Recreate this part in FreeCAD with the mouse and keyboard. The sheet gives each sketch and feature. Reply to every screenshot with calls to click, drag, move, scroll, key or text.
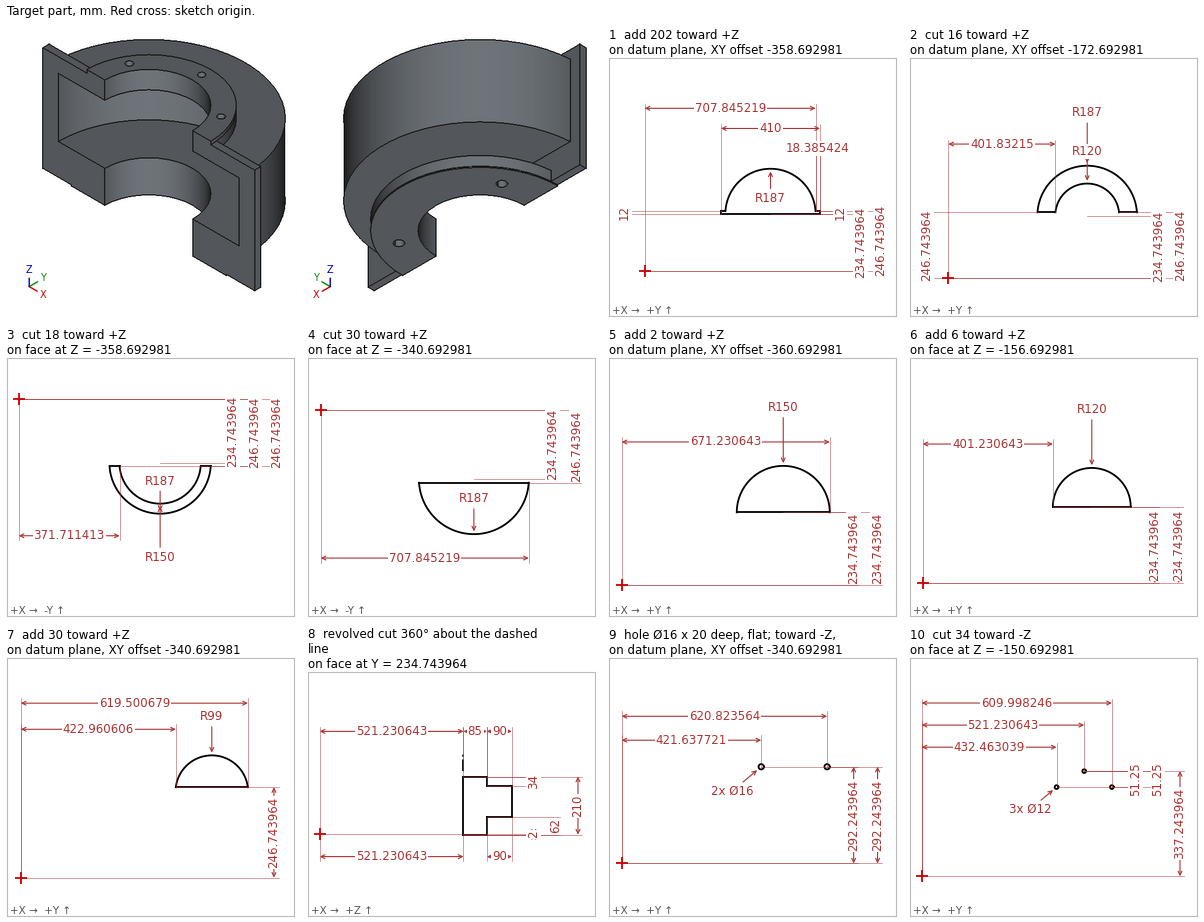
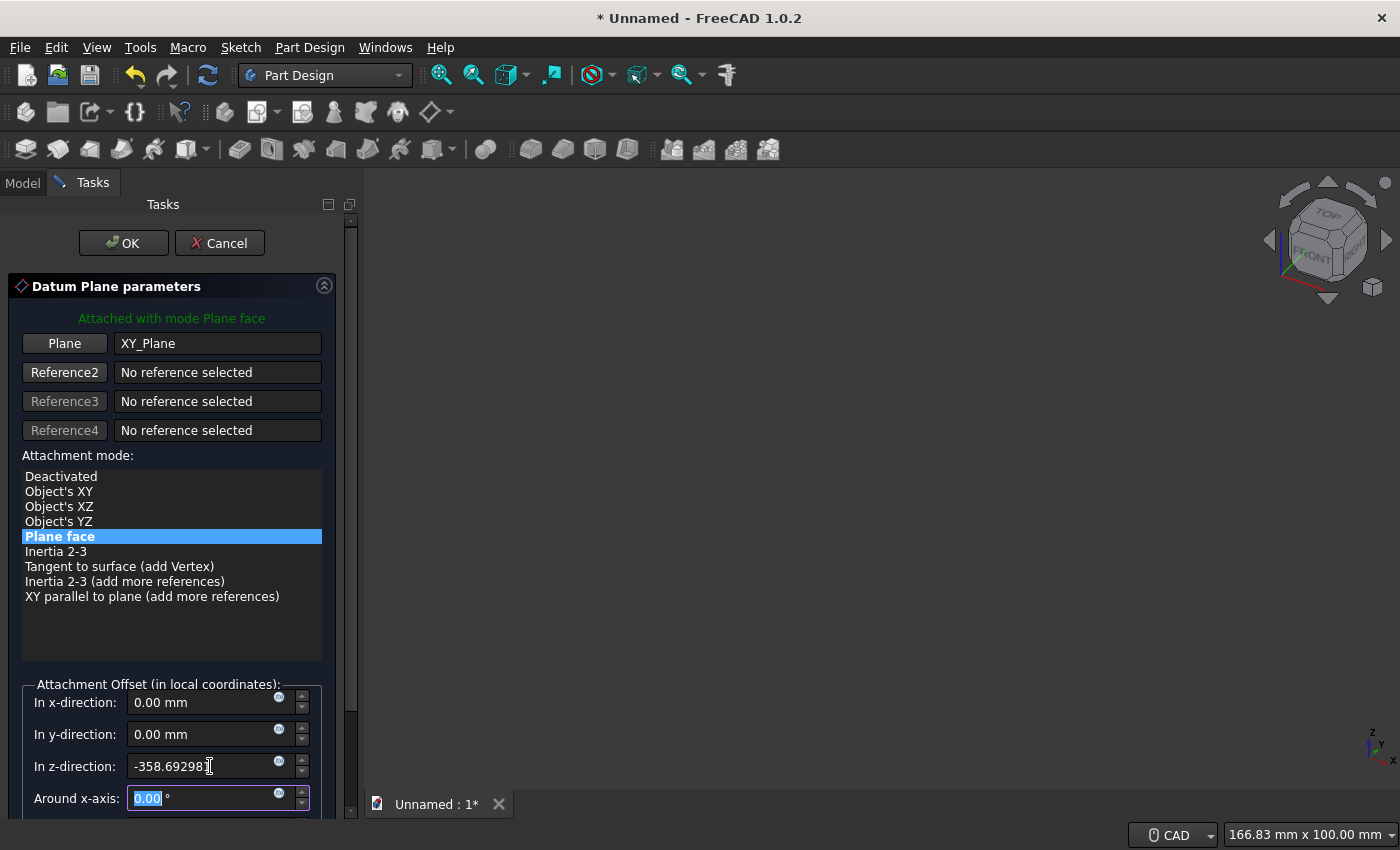
click(124, 243)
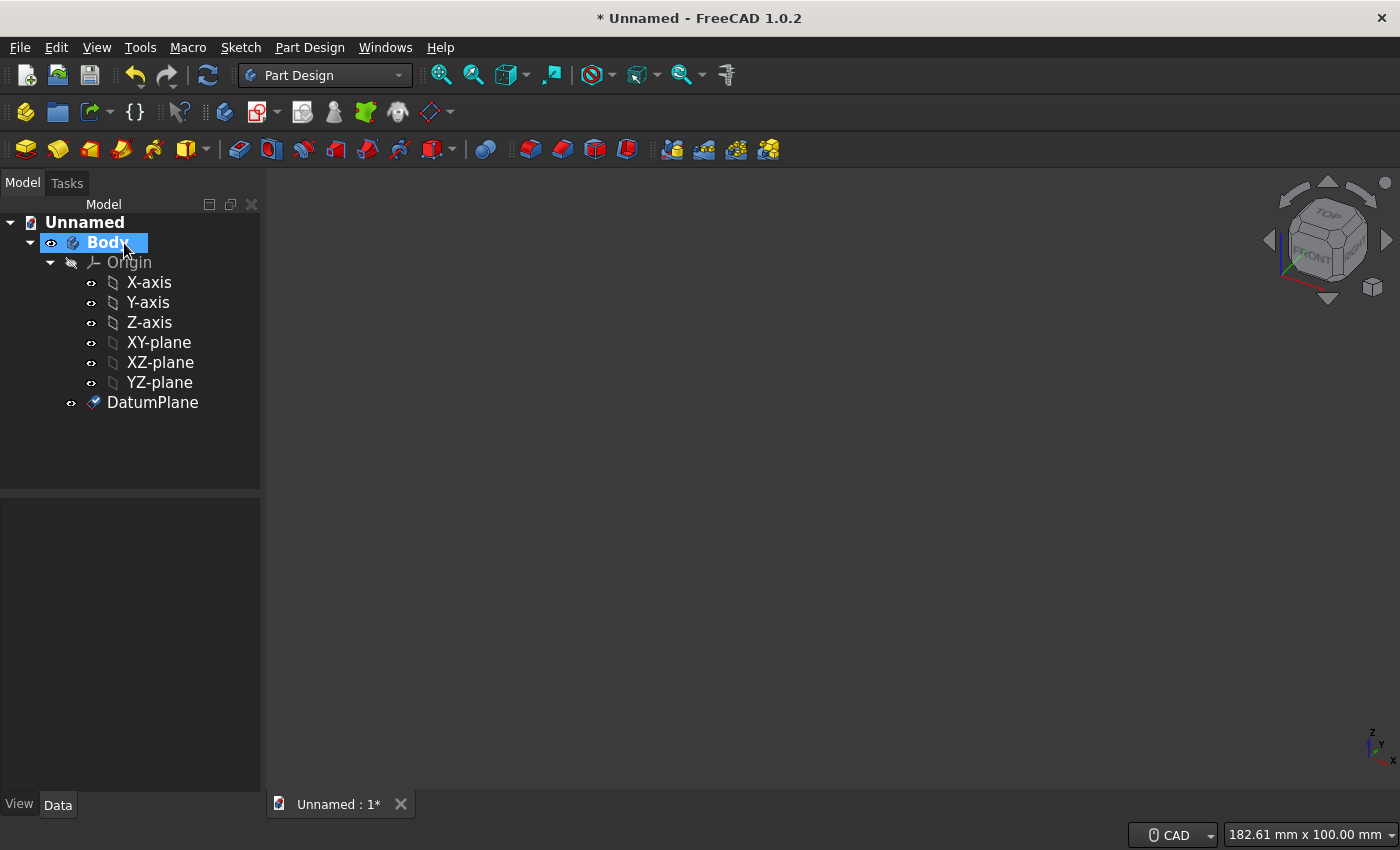
click(116, 403)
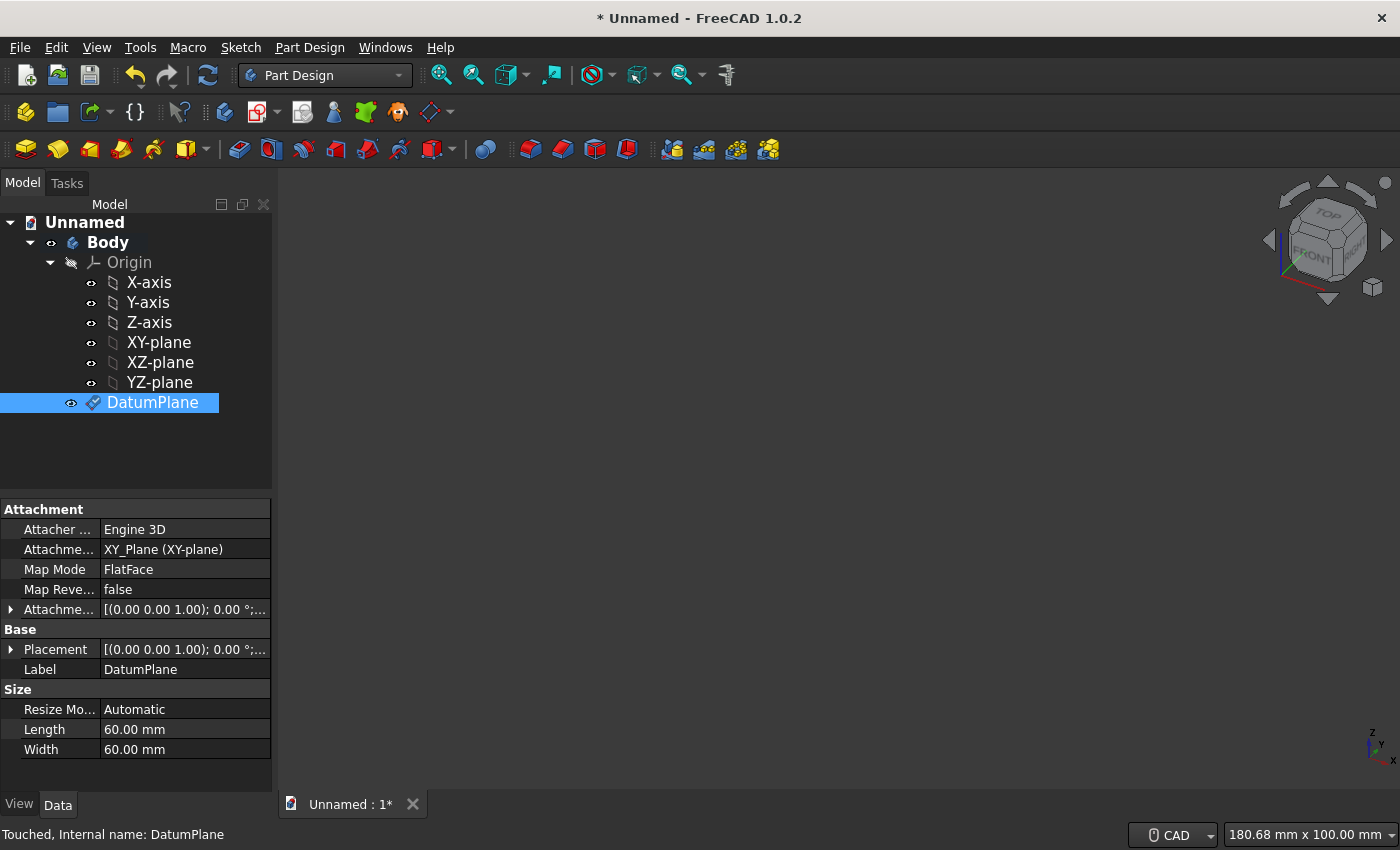
click(258, 112)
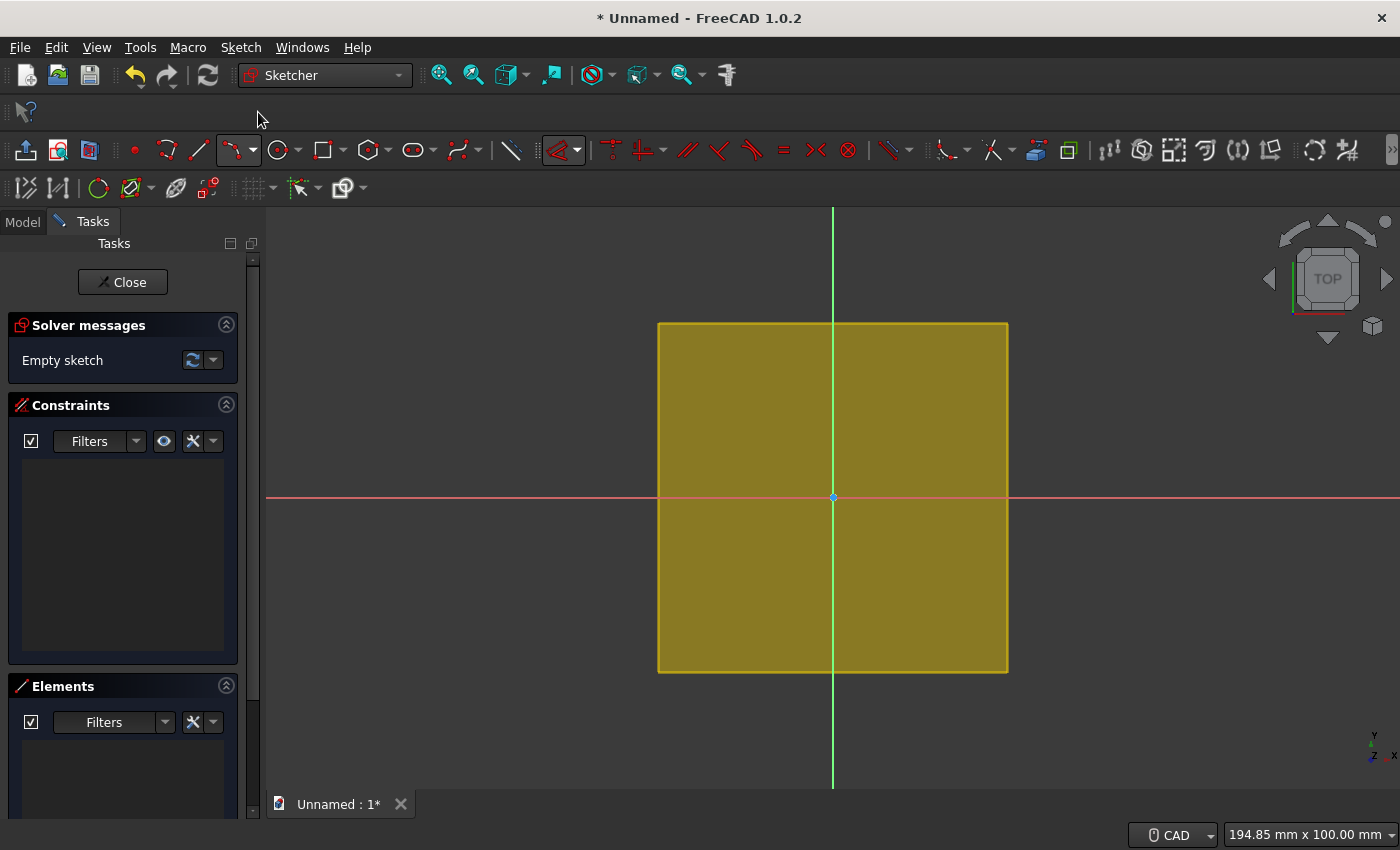
scroll(332, 741, down, 9)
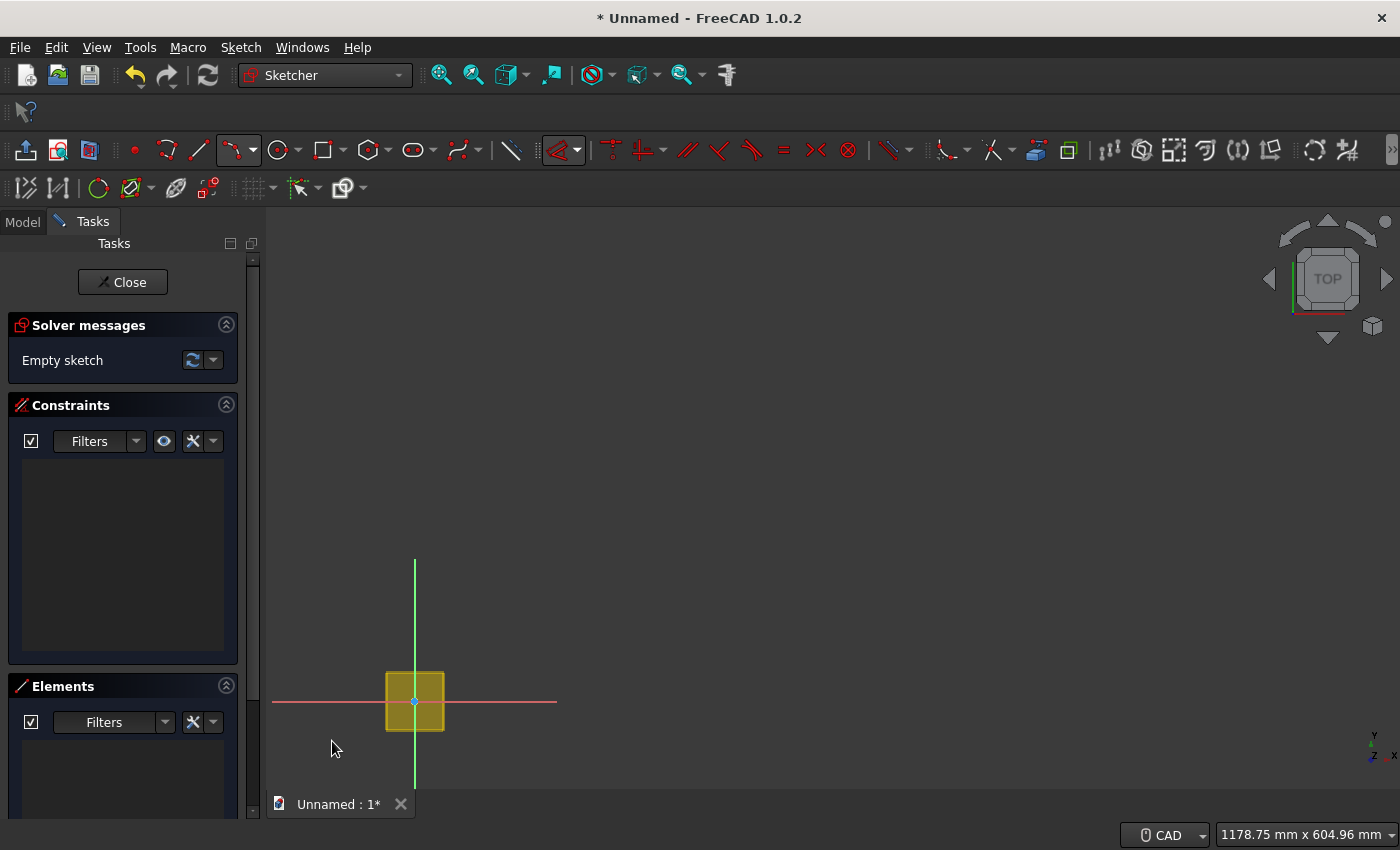
click(168, 150)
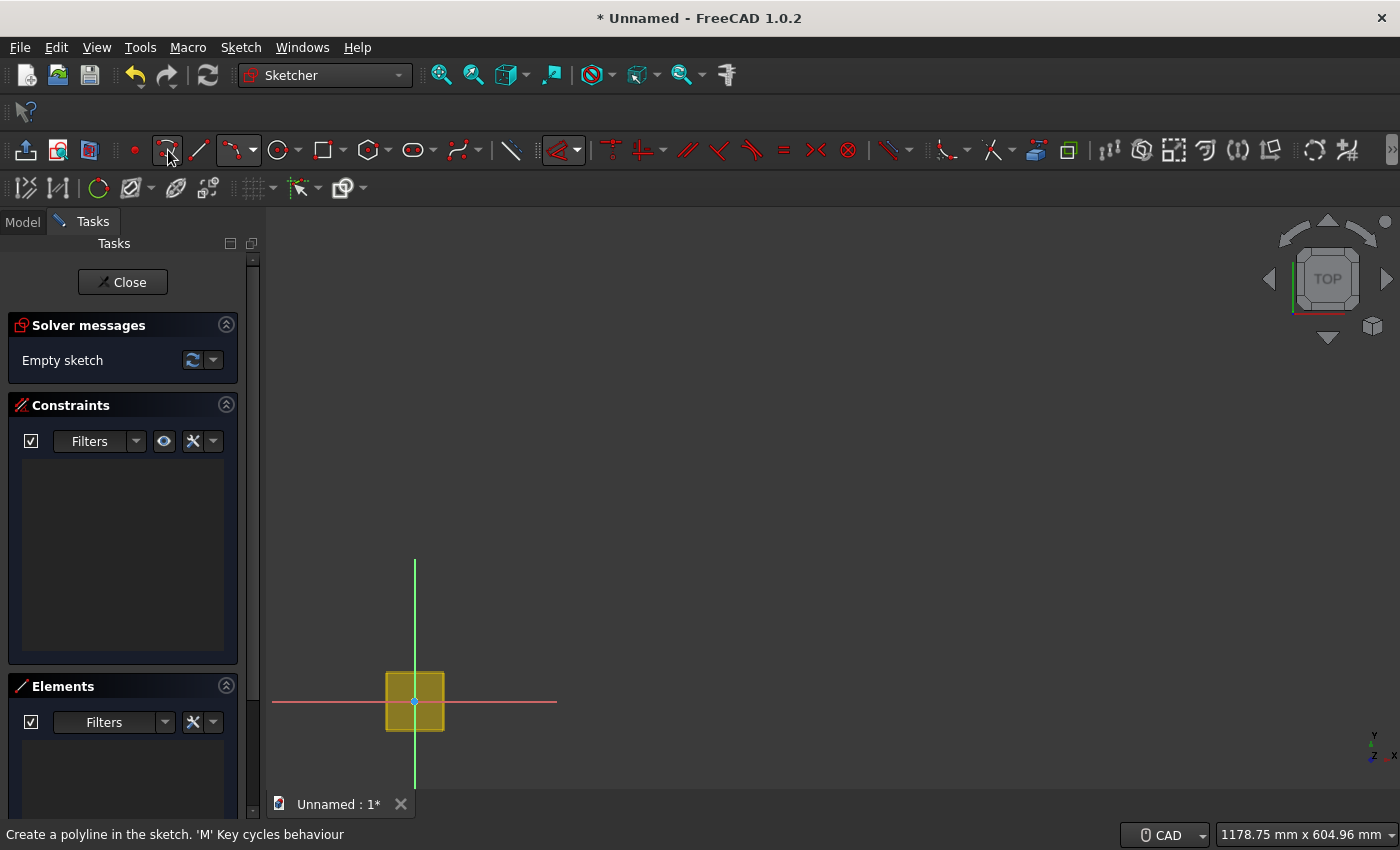
click(1096, 464)
click(1114, 464)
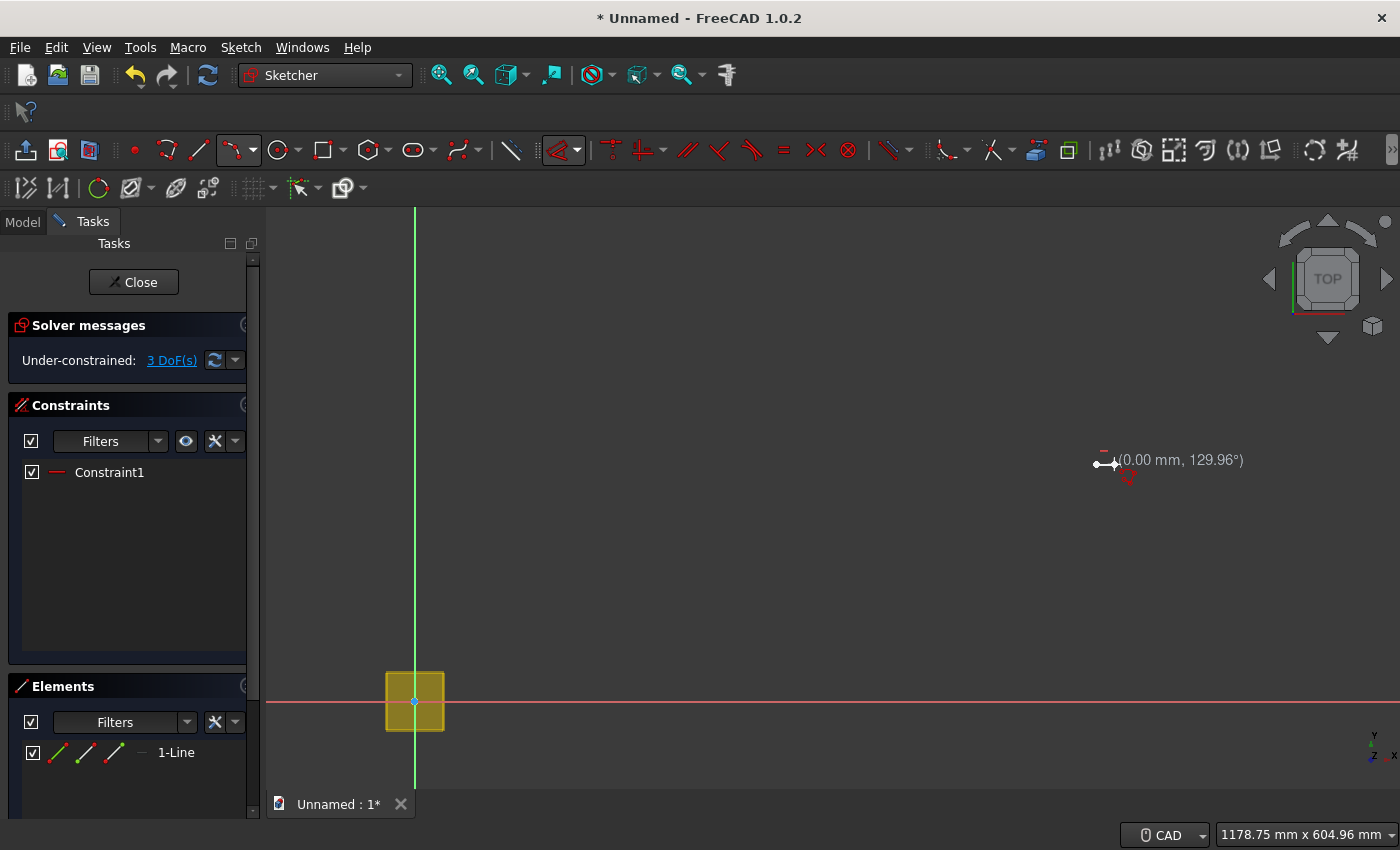
scroll(1114, 476, up, 2)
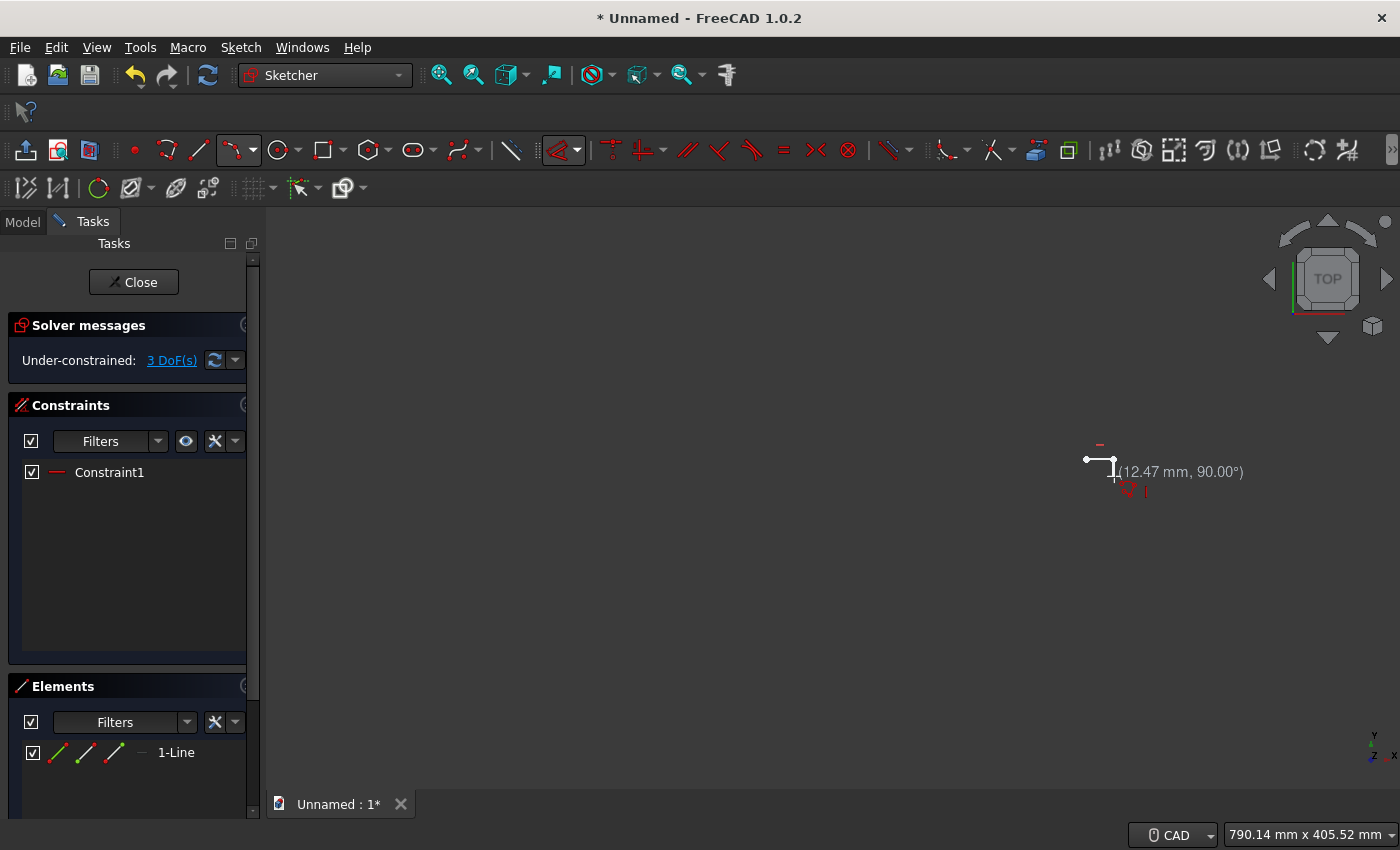
click(1114, 475)
click(524, 475)
click(524, 458)
click(551, 458)
right_click(551, 458)